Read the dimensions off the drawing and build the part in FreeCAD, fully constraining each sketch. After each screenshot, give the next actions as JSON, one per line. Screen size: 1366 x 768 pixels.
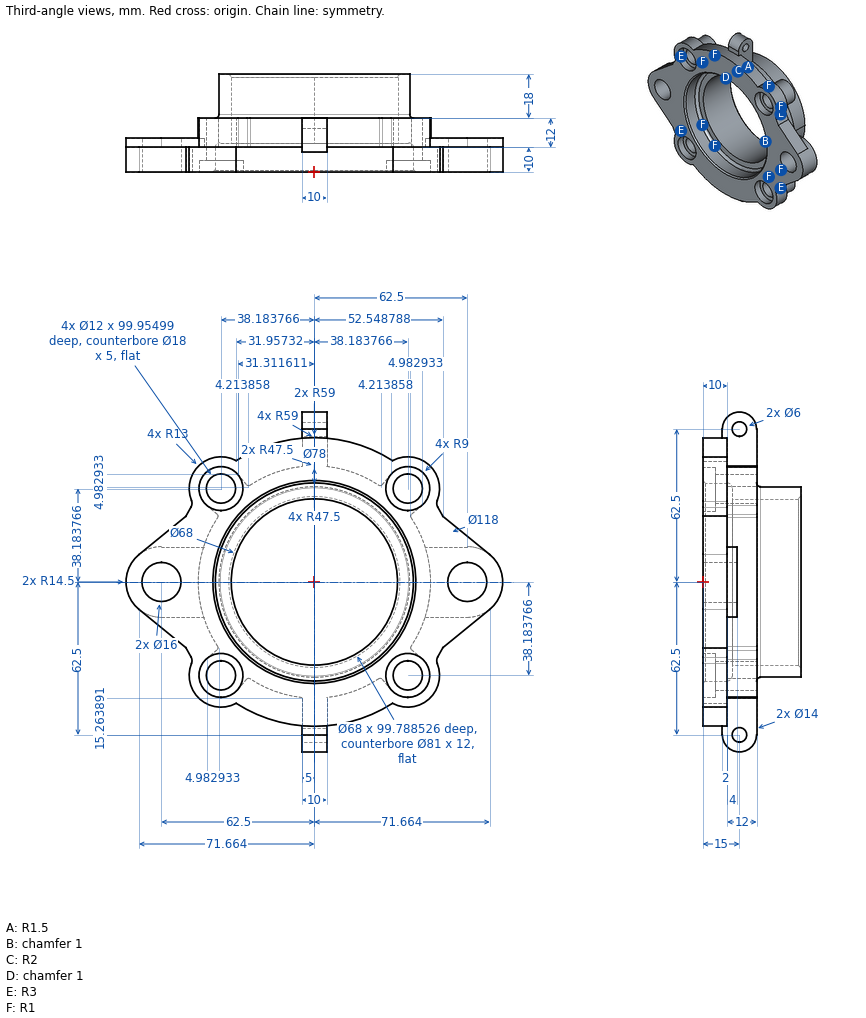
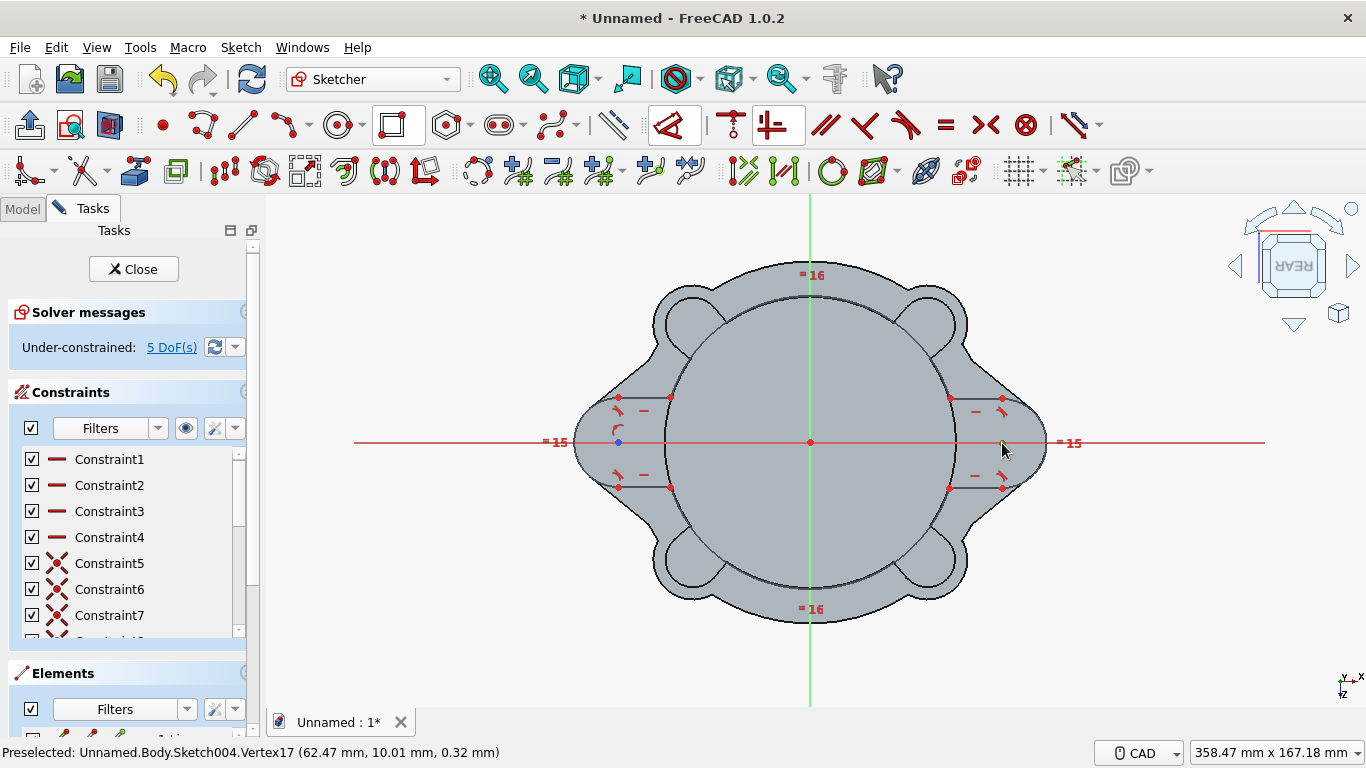
{"action": "left_click", "coordinate": [359, 443]}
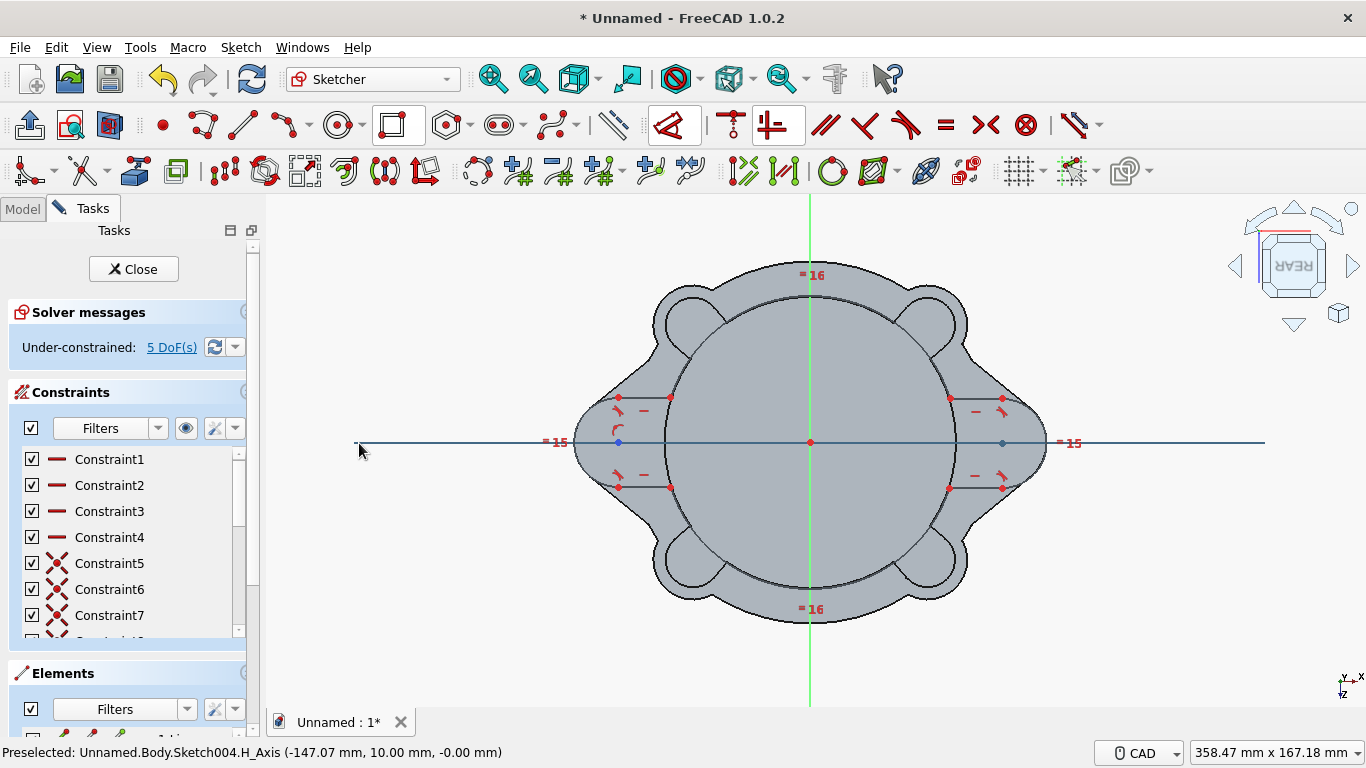
{"action": "left_click", "coordinate": [732, 126]}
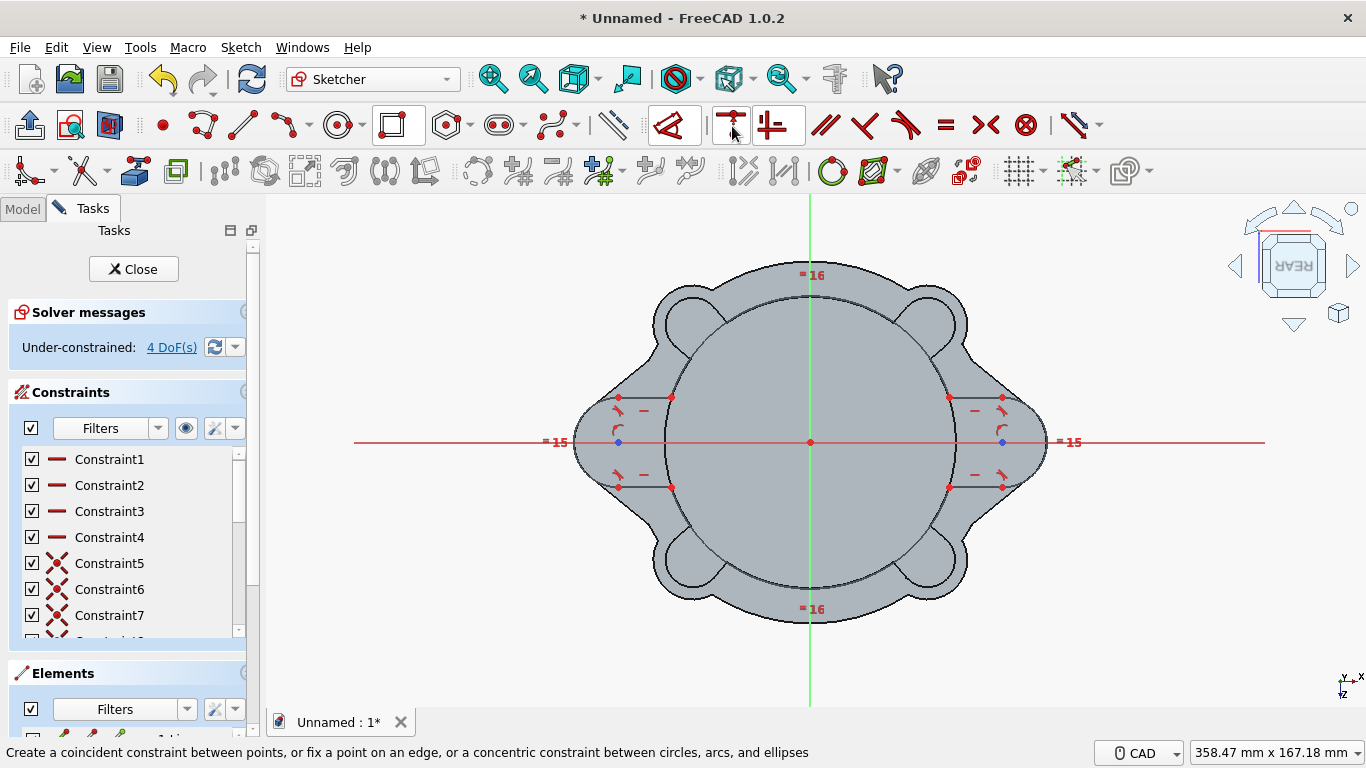
{"action": "left_click", "coordinate": [582, 416]}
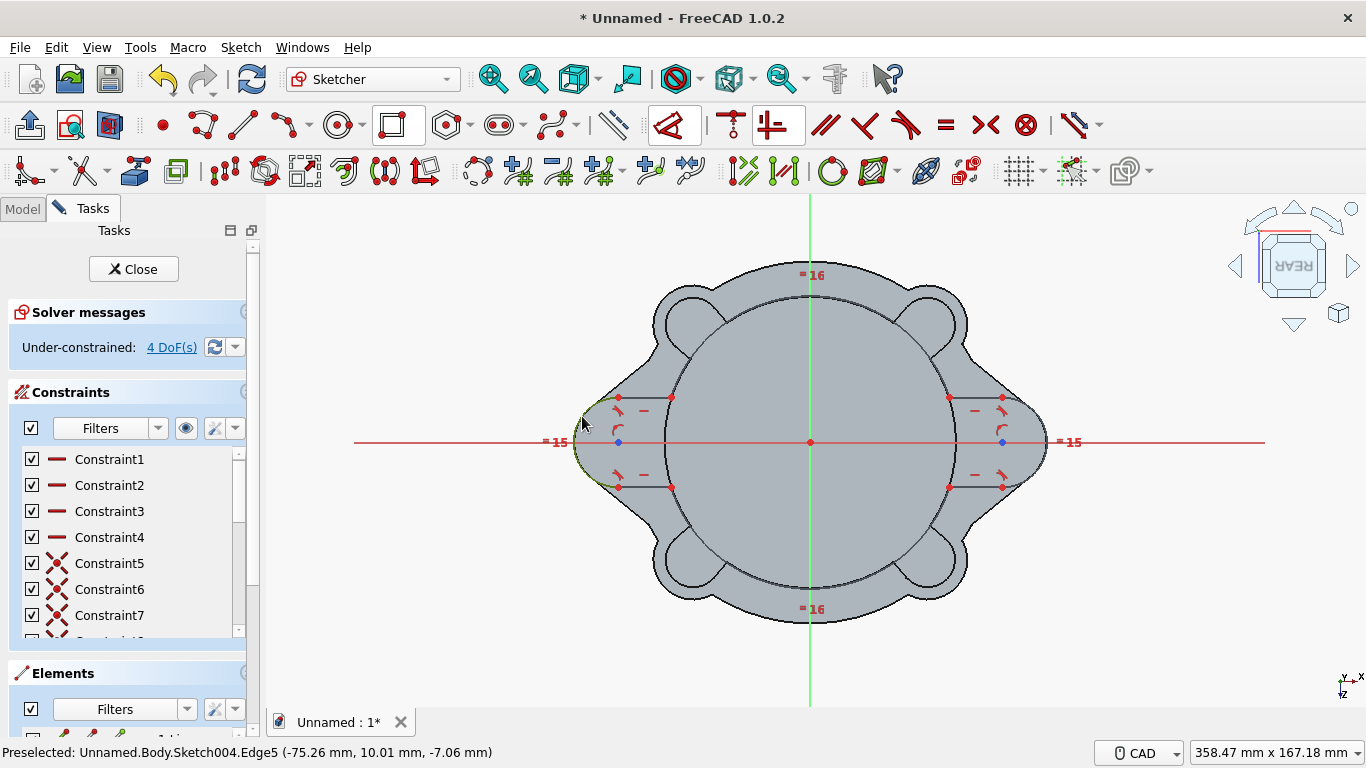
{"action": "key", "text": "k r"}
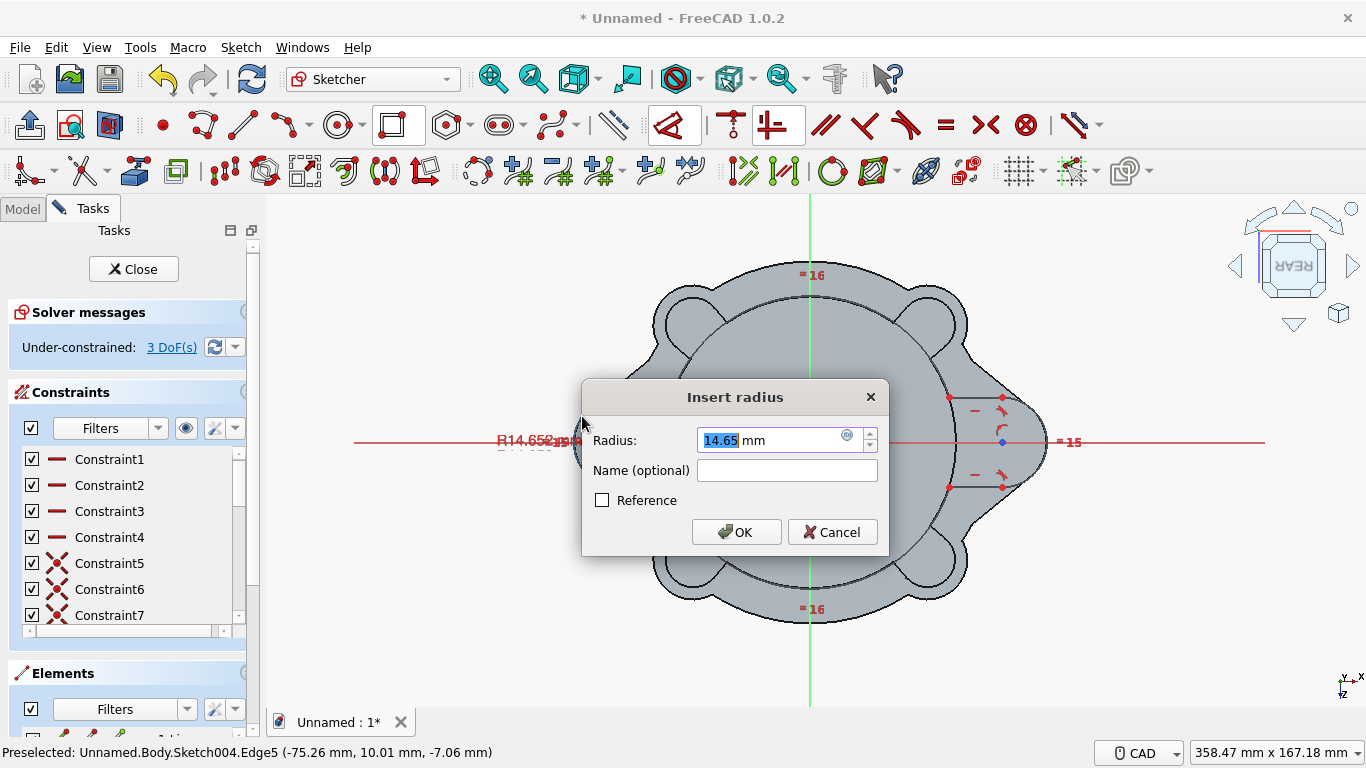
{"action": "type", "text": "14.5"}
{"action": "key", "text": "Return"}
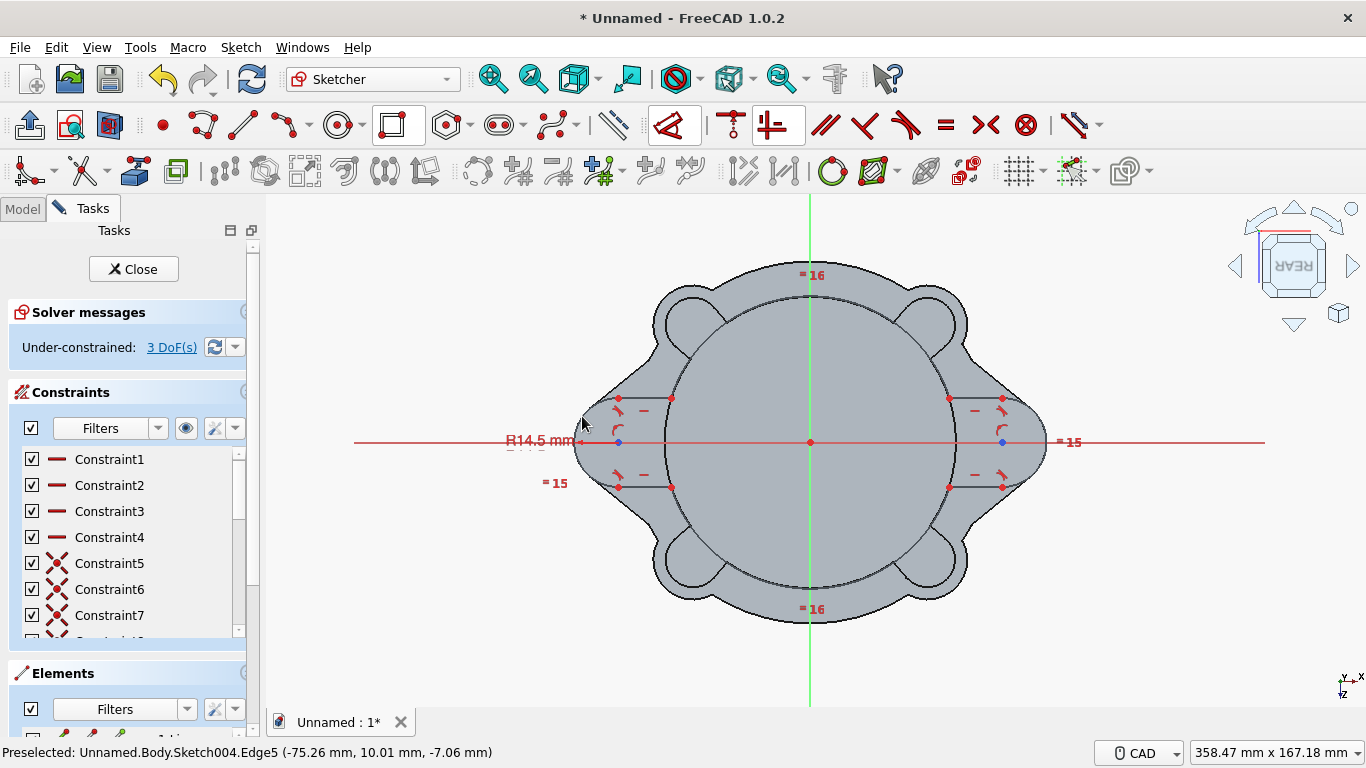
{"action": "left_click", "coordinate": [740, 571]}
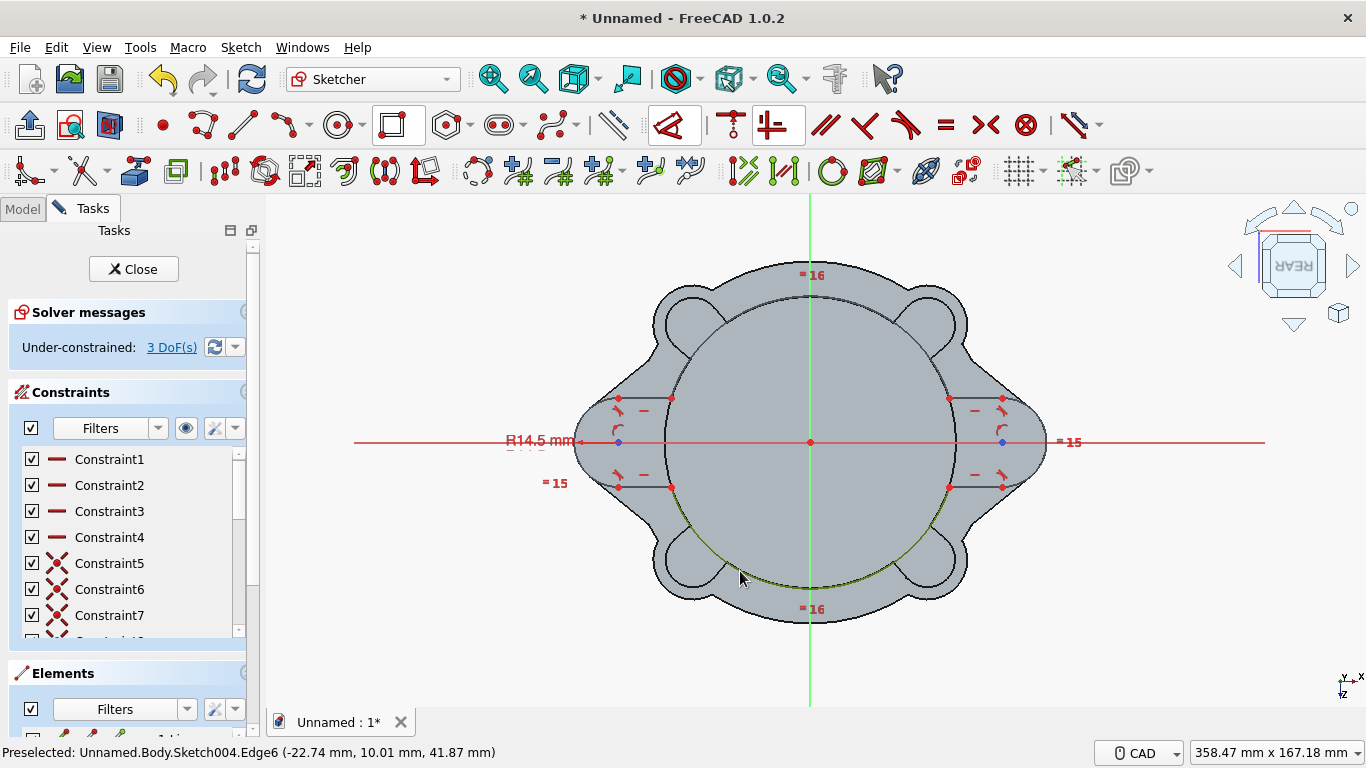
{"action": "left_click", "coordinate": [696, 126]}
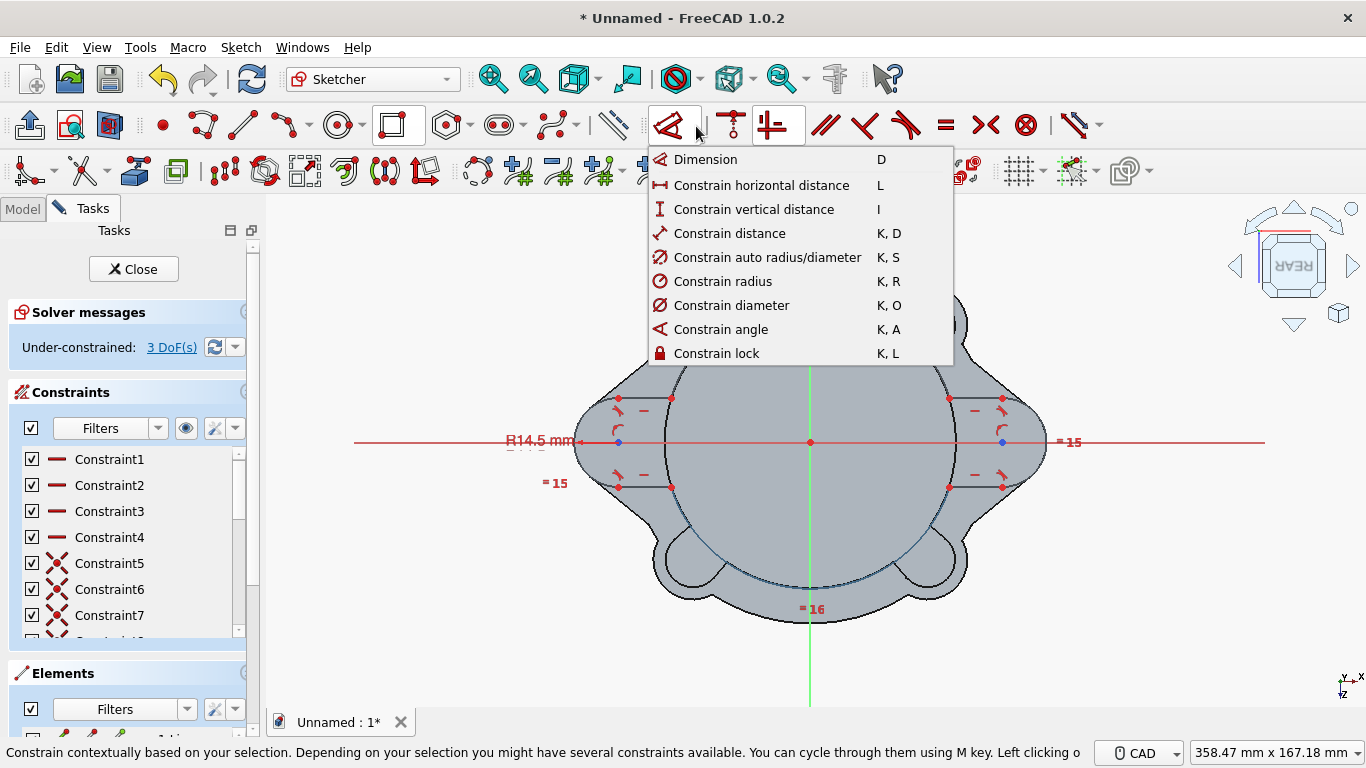
{"action": "left_click", "coordinate": [801, 281]}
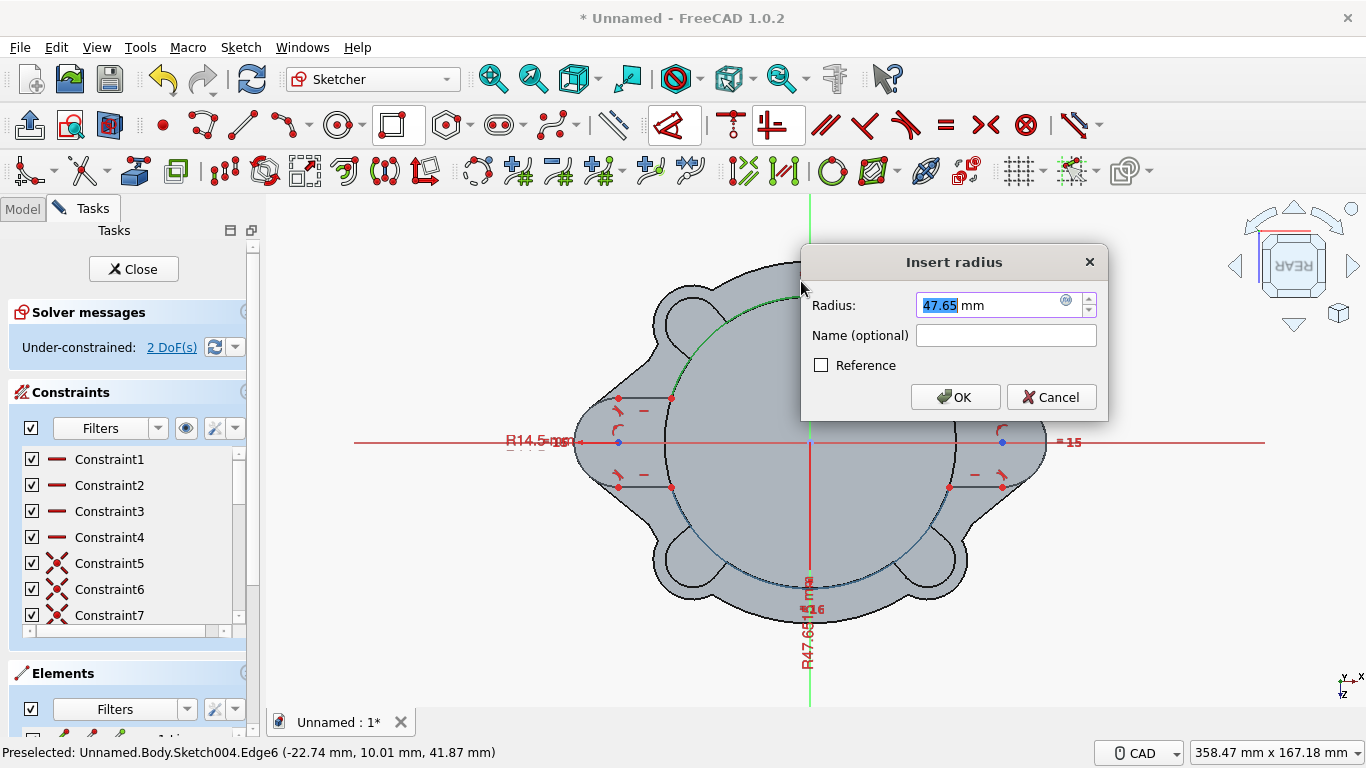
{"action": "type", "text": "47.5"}
{"action": "key", "text": "Return"}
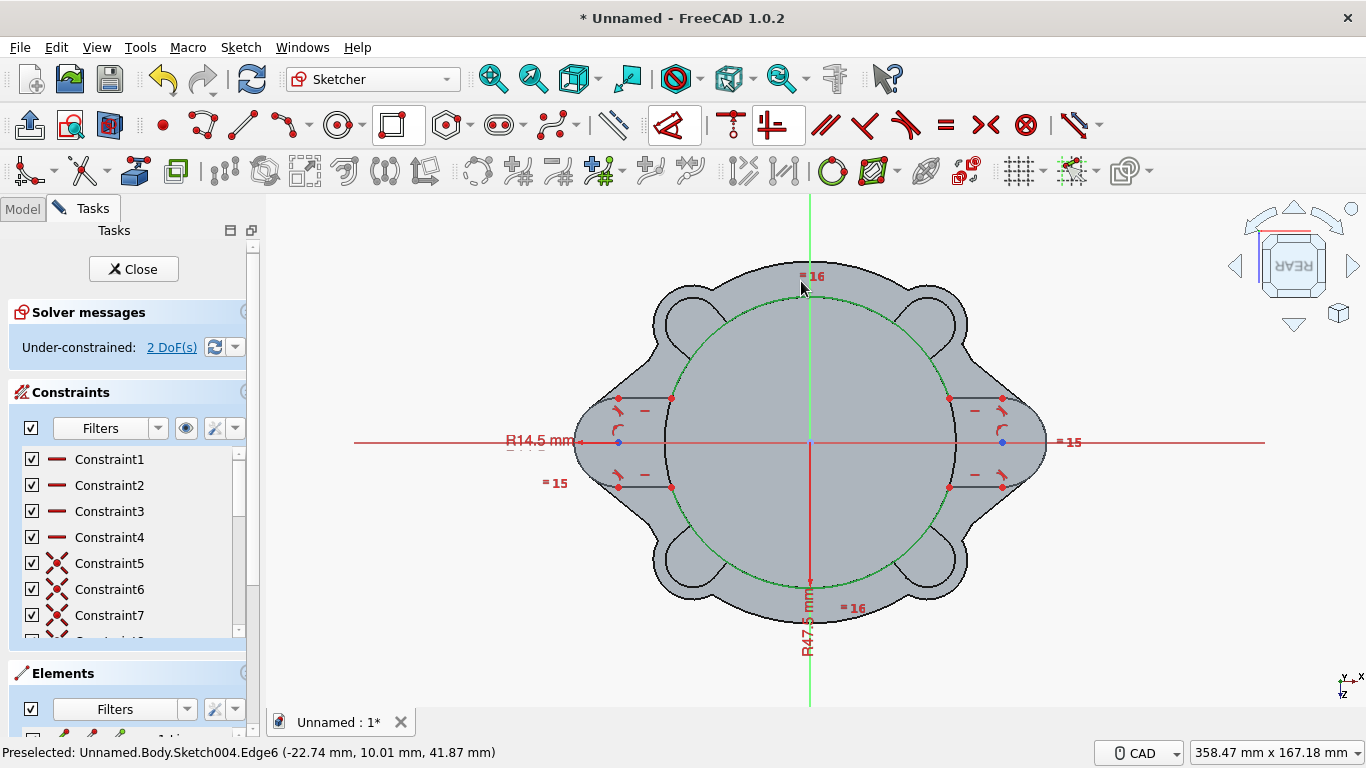
{"action": "left_click", "coordinate": [619, 398]}